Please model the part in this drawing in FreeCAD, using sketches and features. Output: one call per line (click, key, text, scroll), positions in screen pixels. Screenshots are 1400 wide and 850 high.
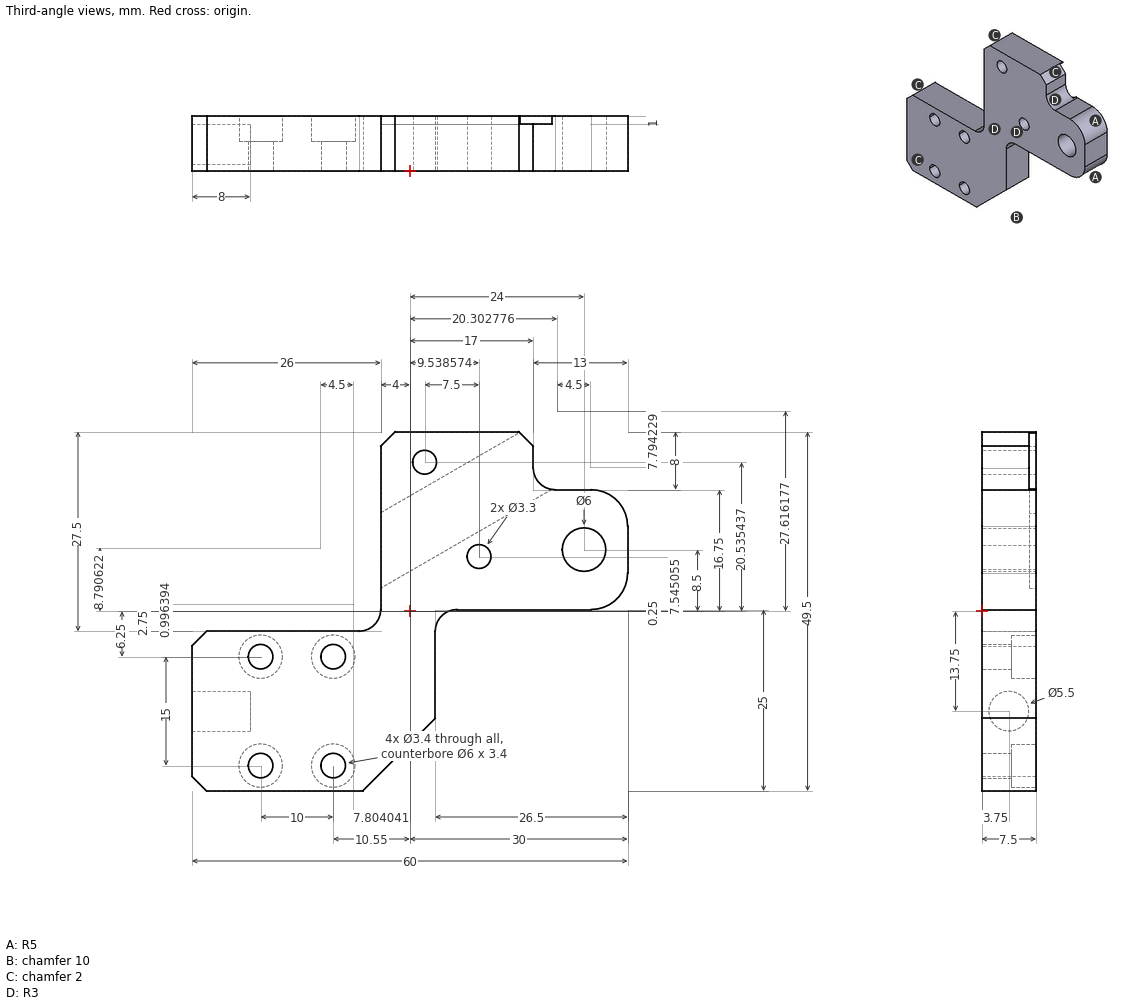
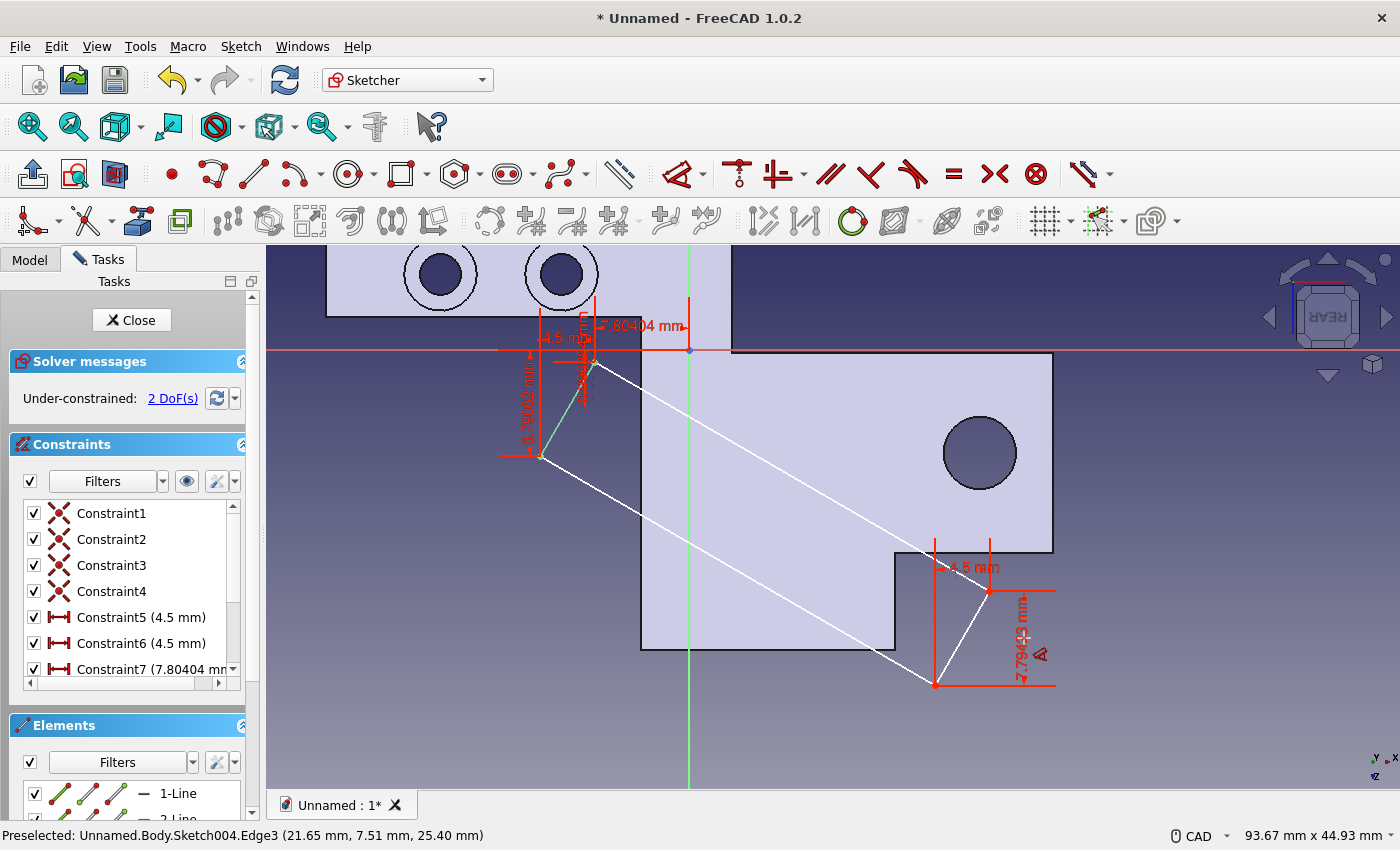
click(935, 686)
click(812, 720)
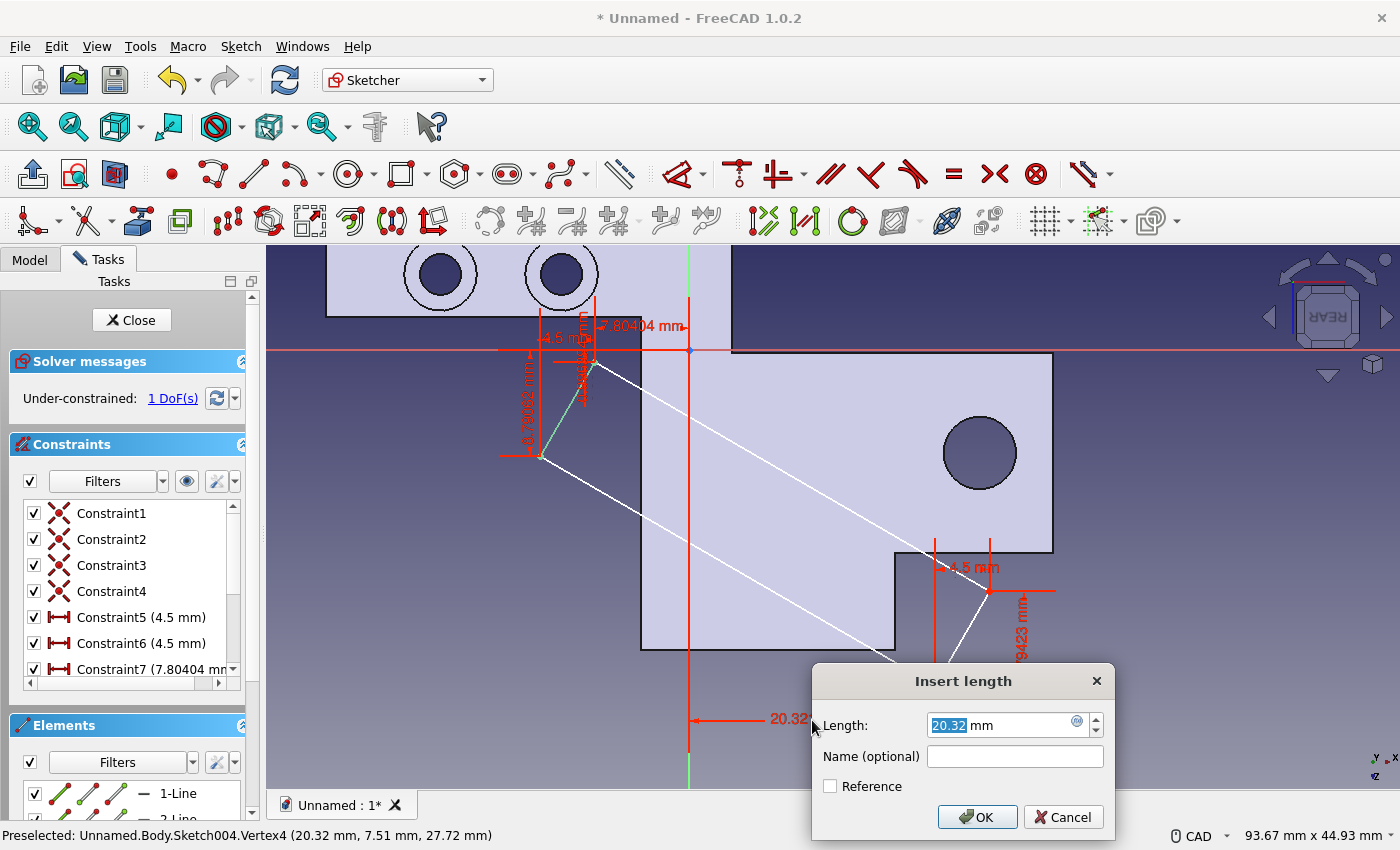
text(20.302776)
key(Return)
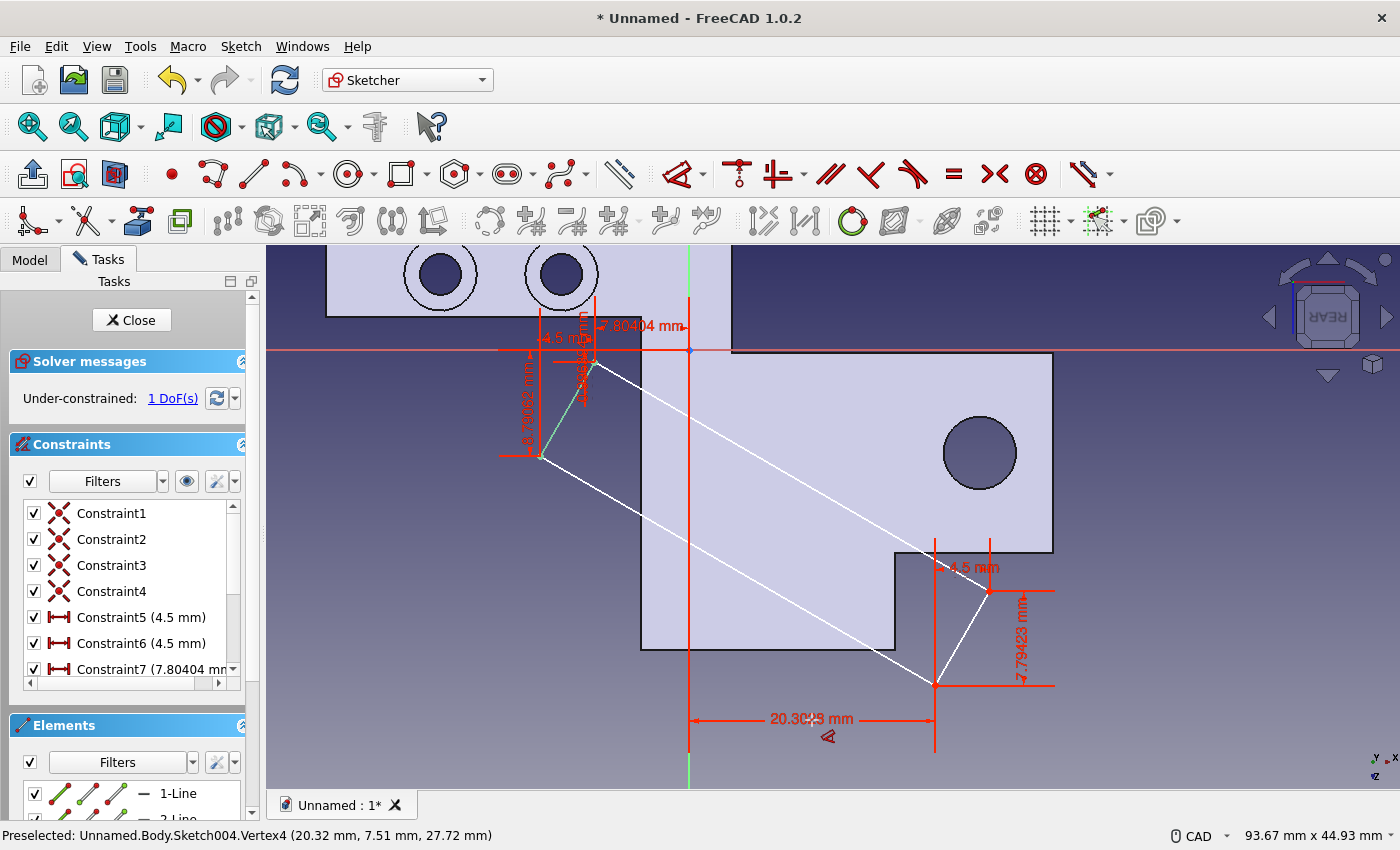
click(935, 686)
click(969, 518)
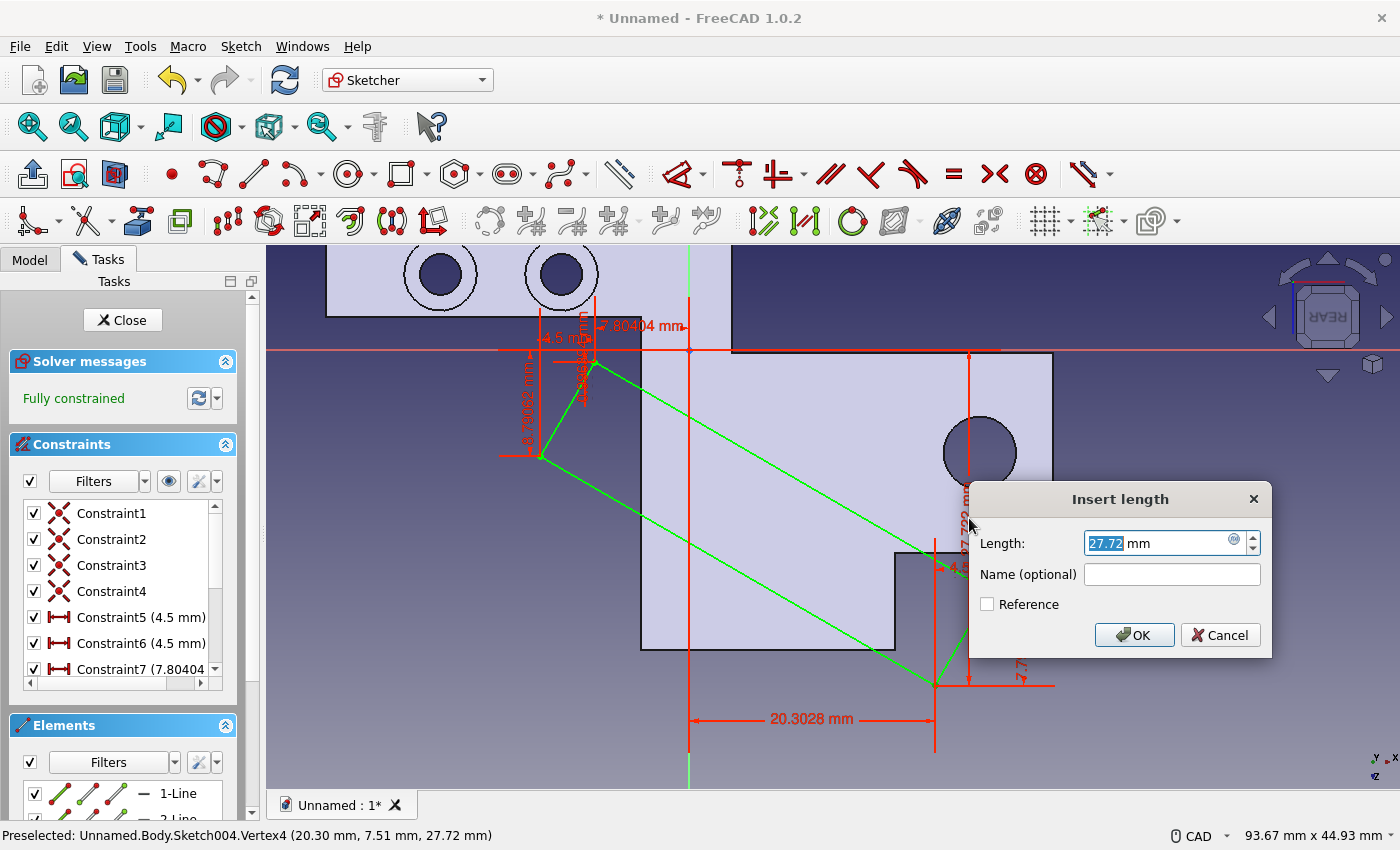
text(27.616177)
key(Return)
key(Escape)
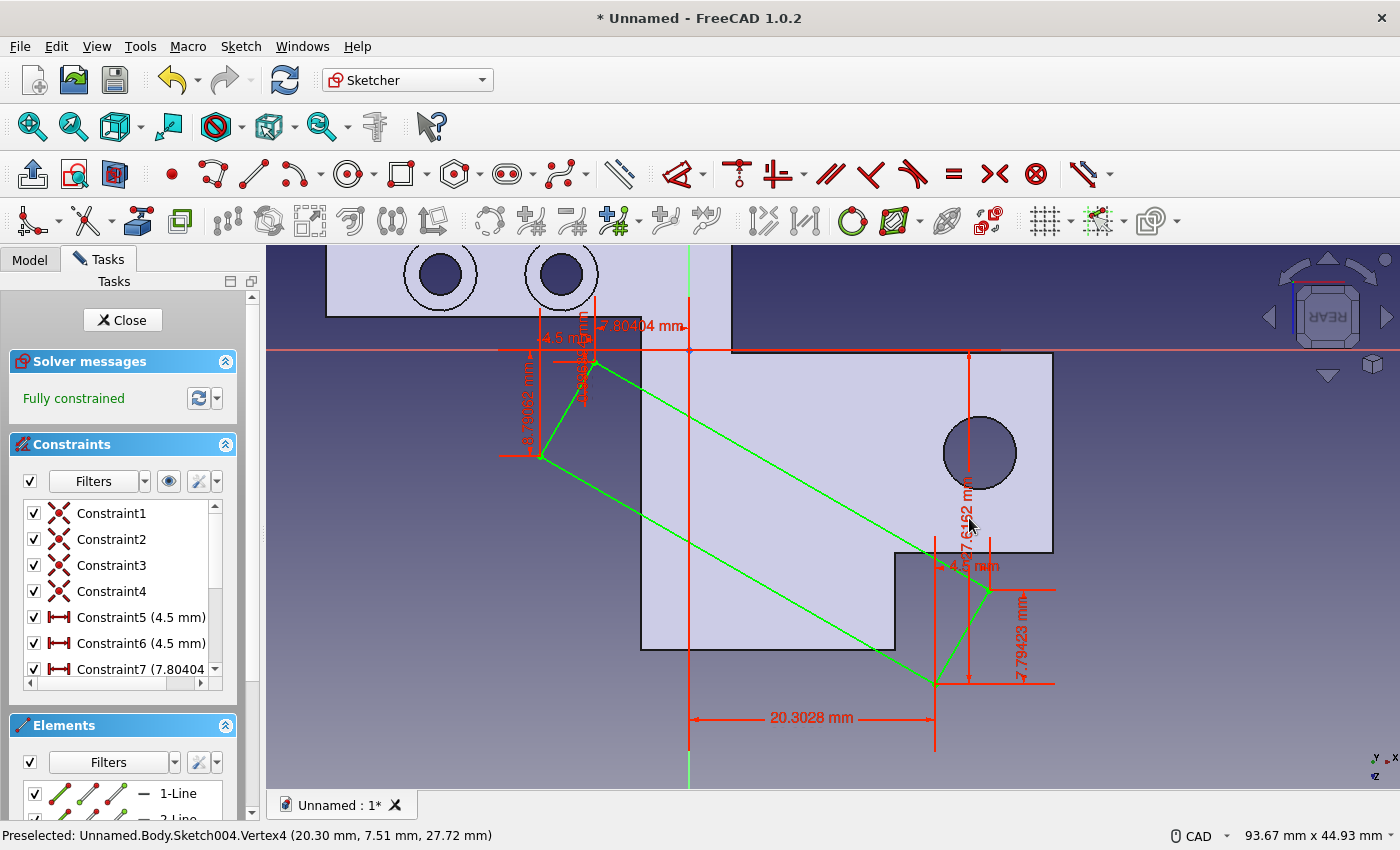
click(123, 320)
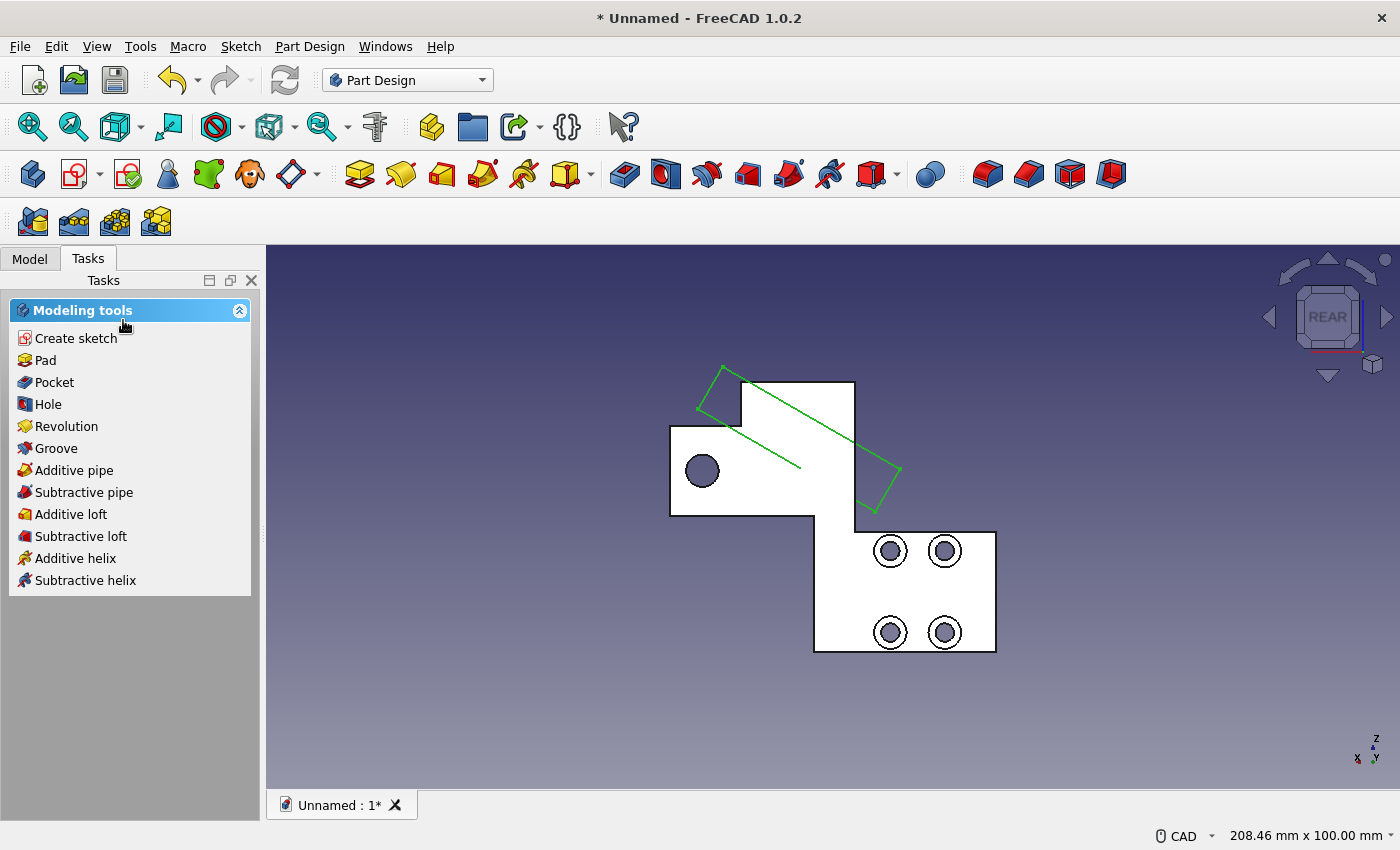
click(625, 174)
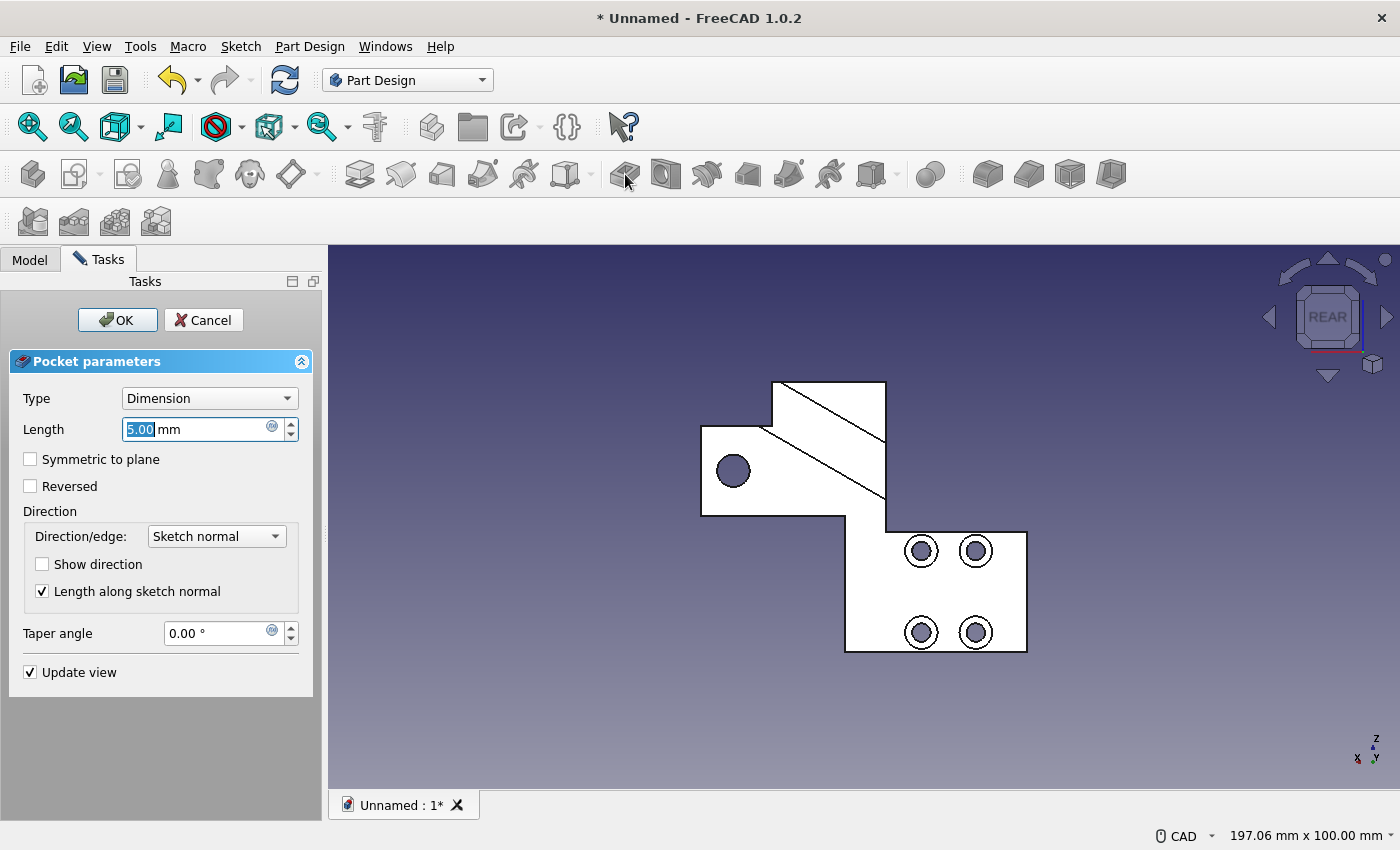
text(1)
key(Tab)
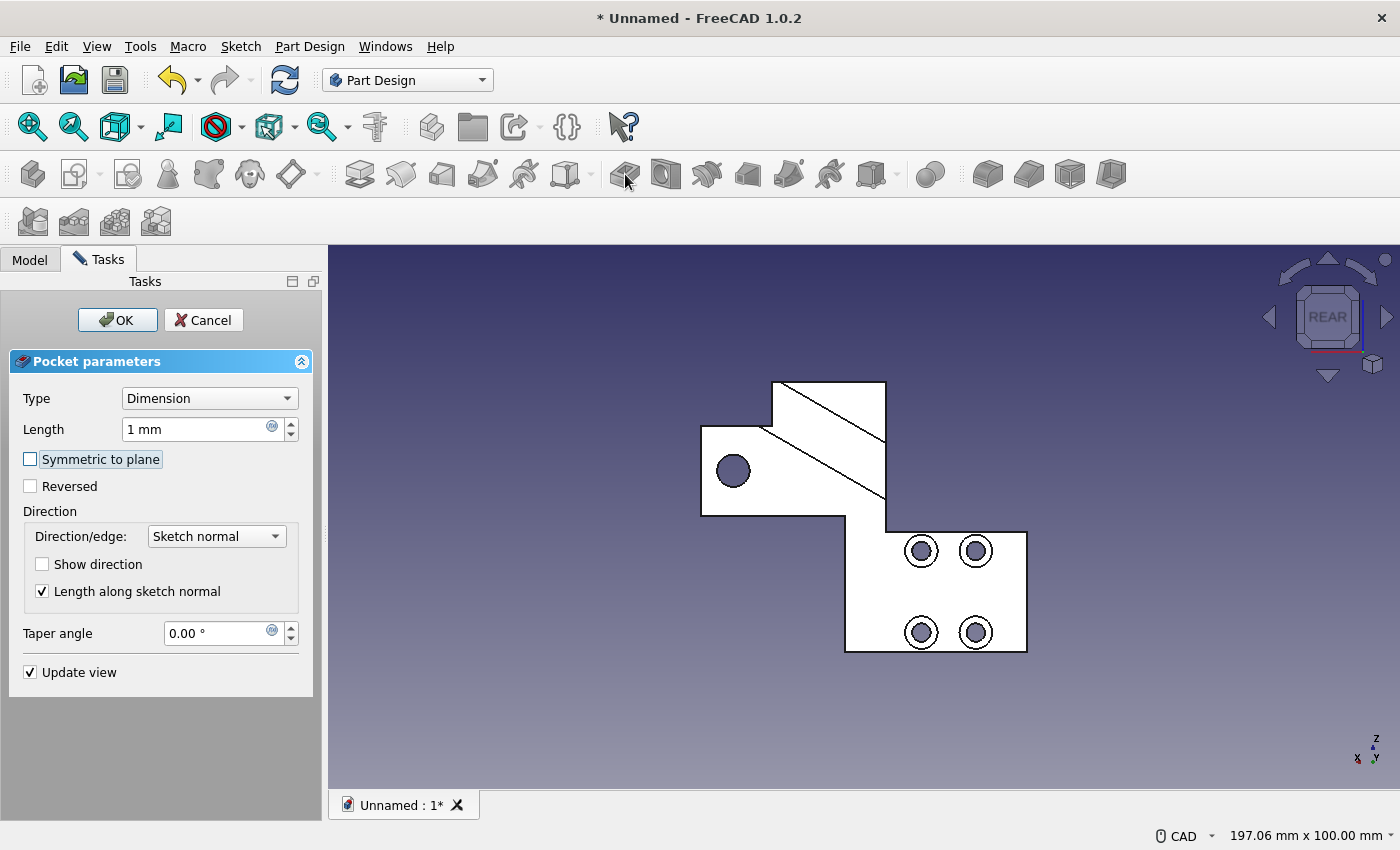
click(118, 320)